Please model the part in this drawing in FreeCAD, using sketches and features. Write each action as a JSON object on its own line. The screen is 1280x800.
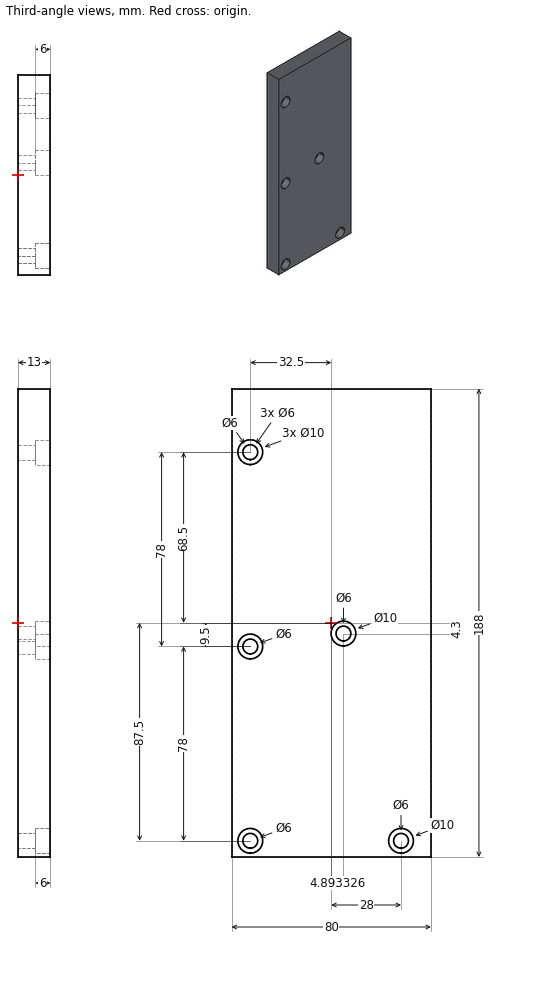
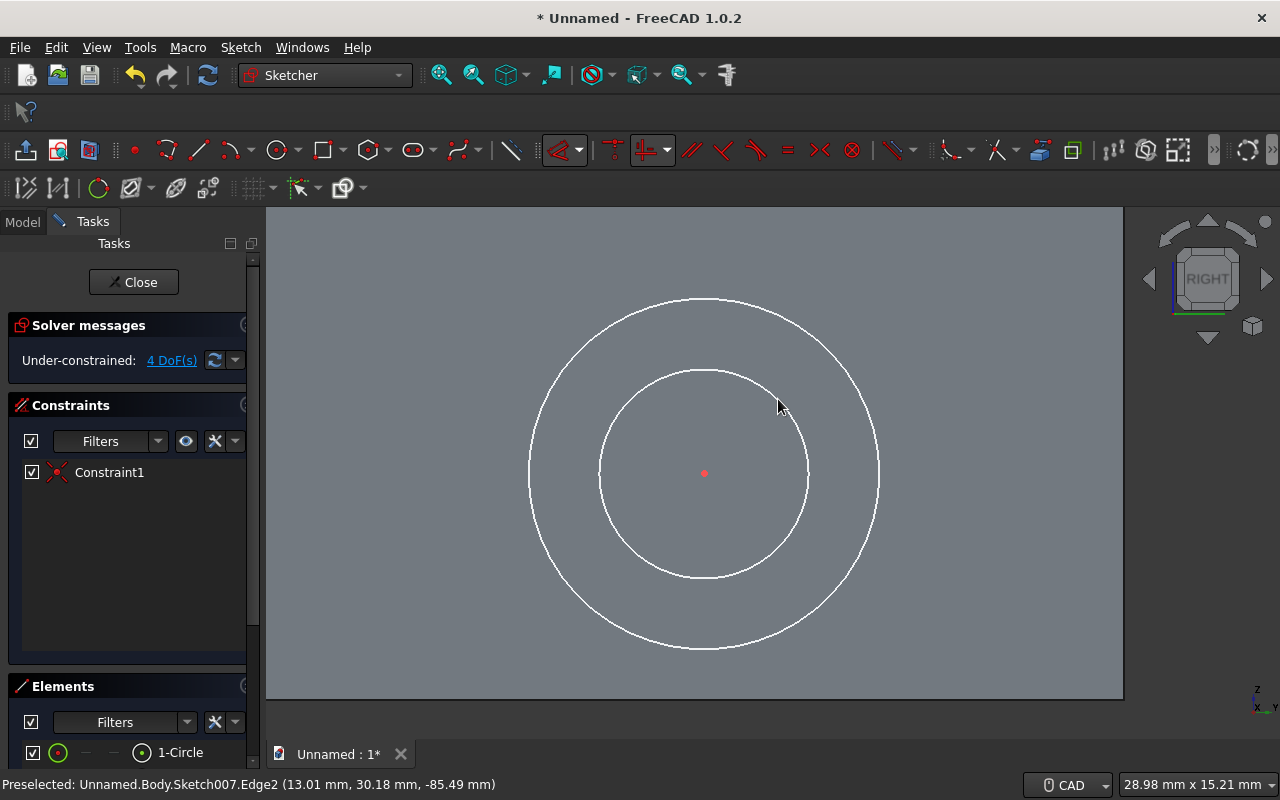
{"action": "left_click", "coordinate": [828, 350]}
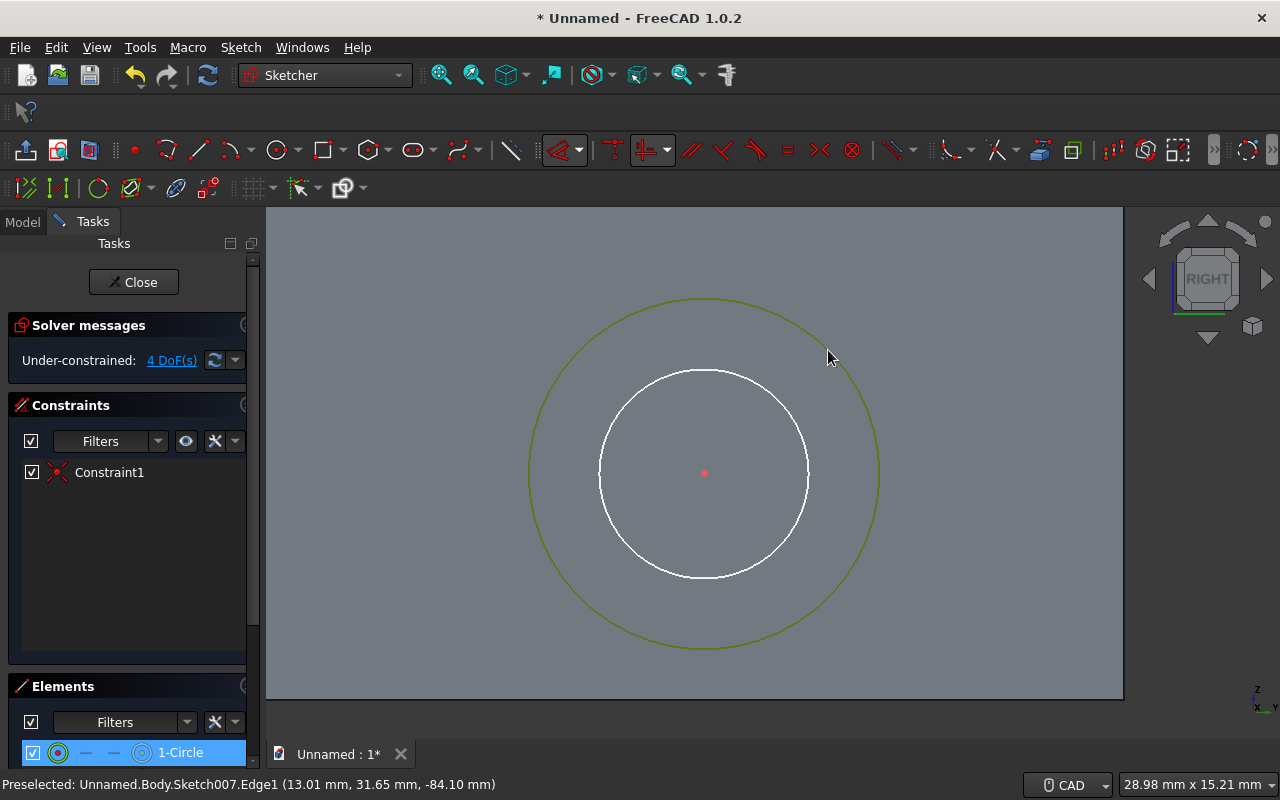
{"action": "left_click", "coordinate": [582, 150]}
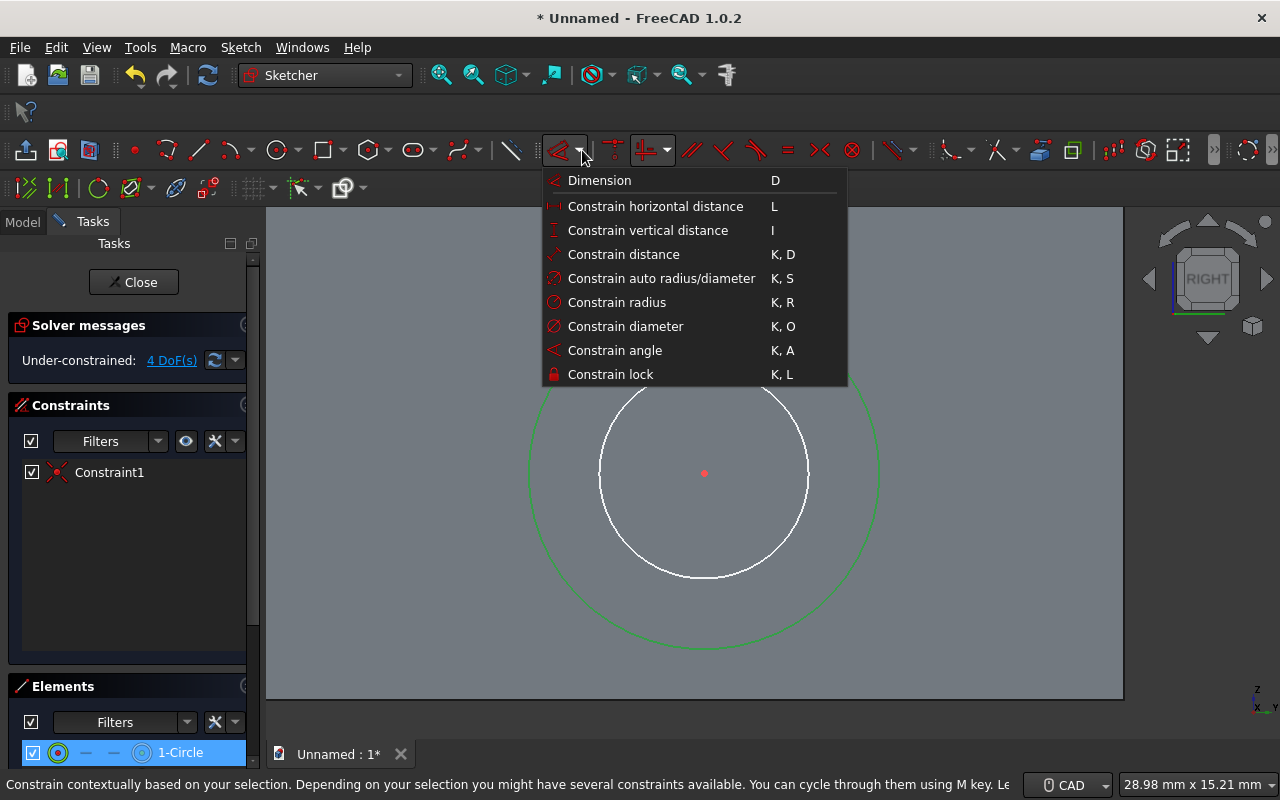
{"action": "left_click", "coordinate": [695, 326]}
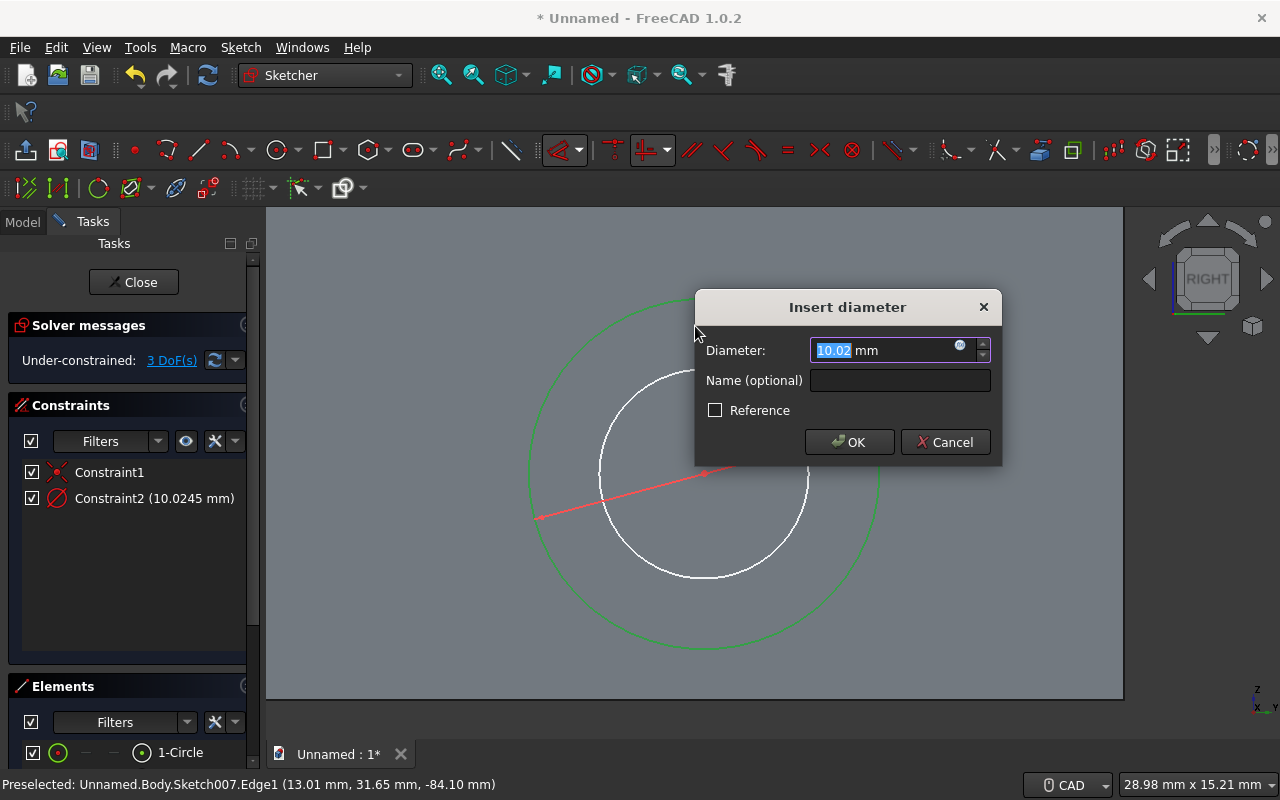
{"action": "type", "text": "10"}
{"action": "key", "text": "Return"}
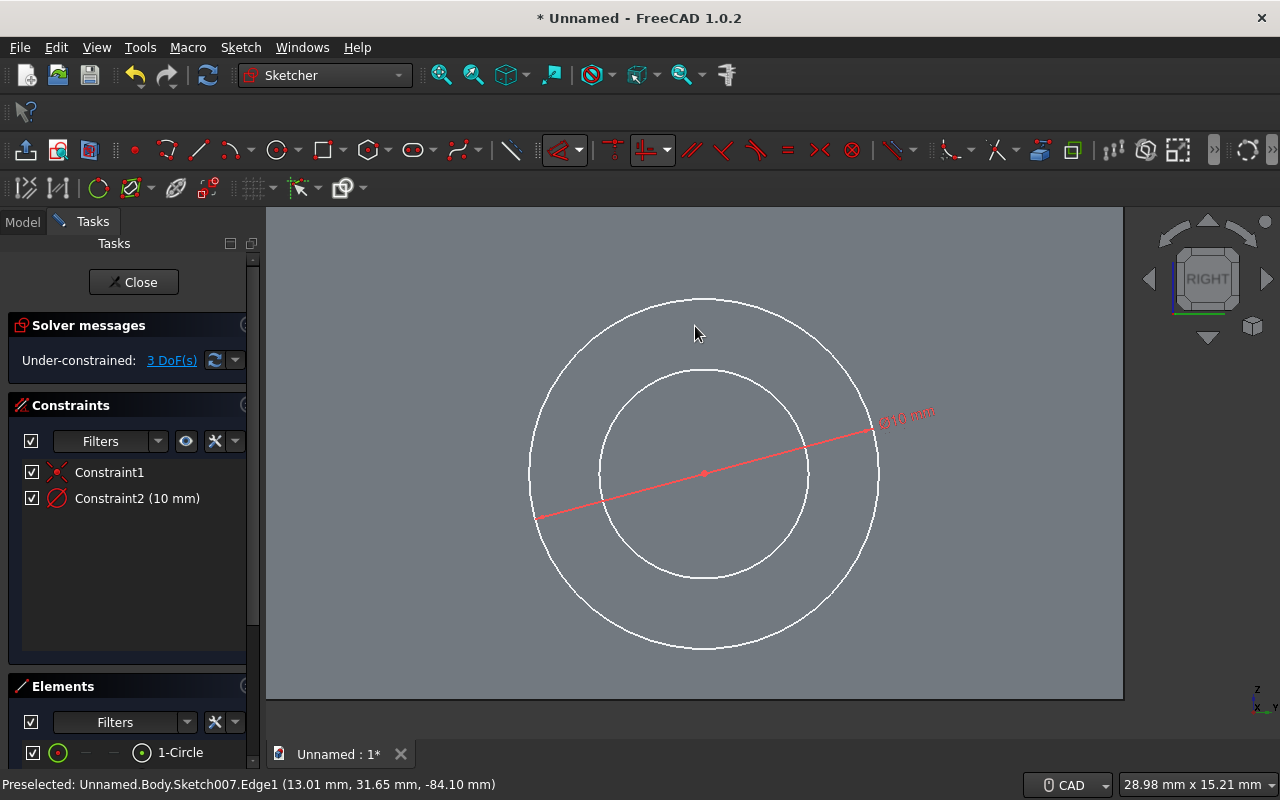
{"action": "left_click", "coordinate": [778, 400]}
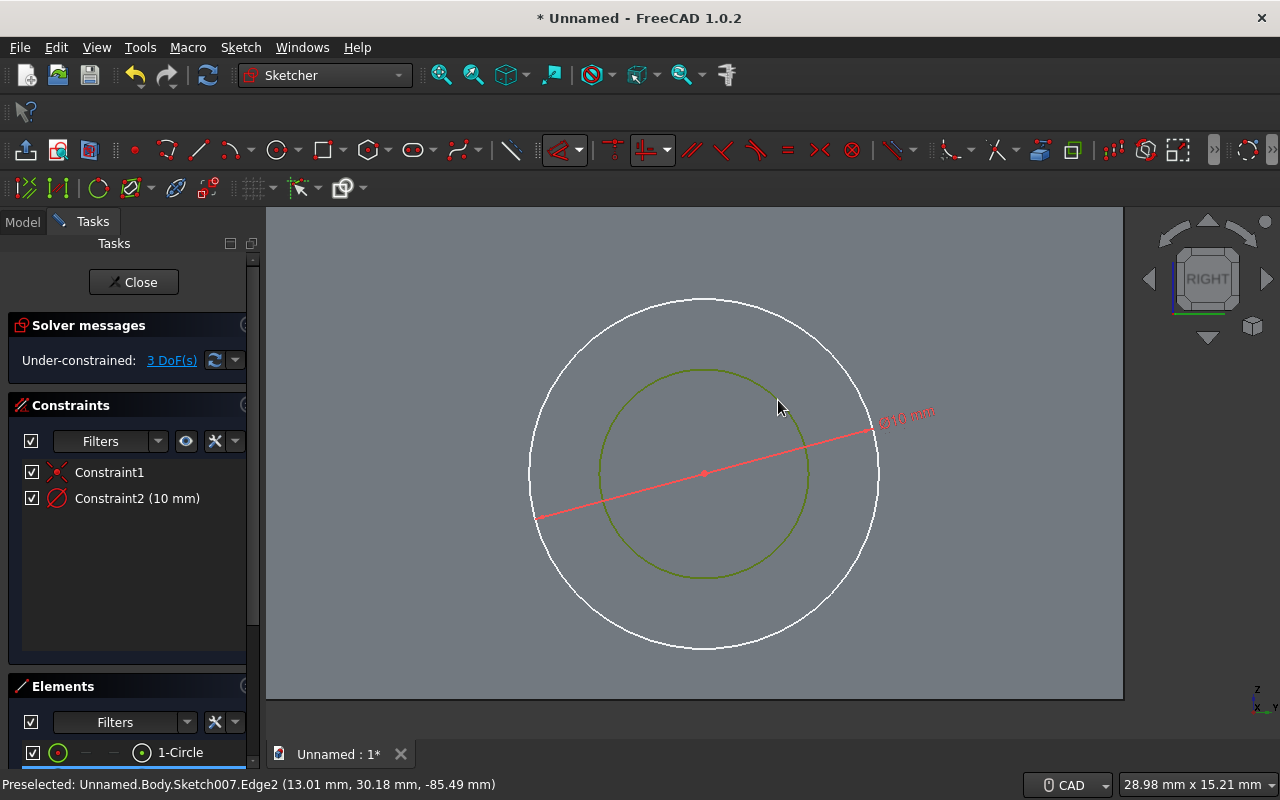
{"action": "key", "text": "k o"}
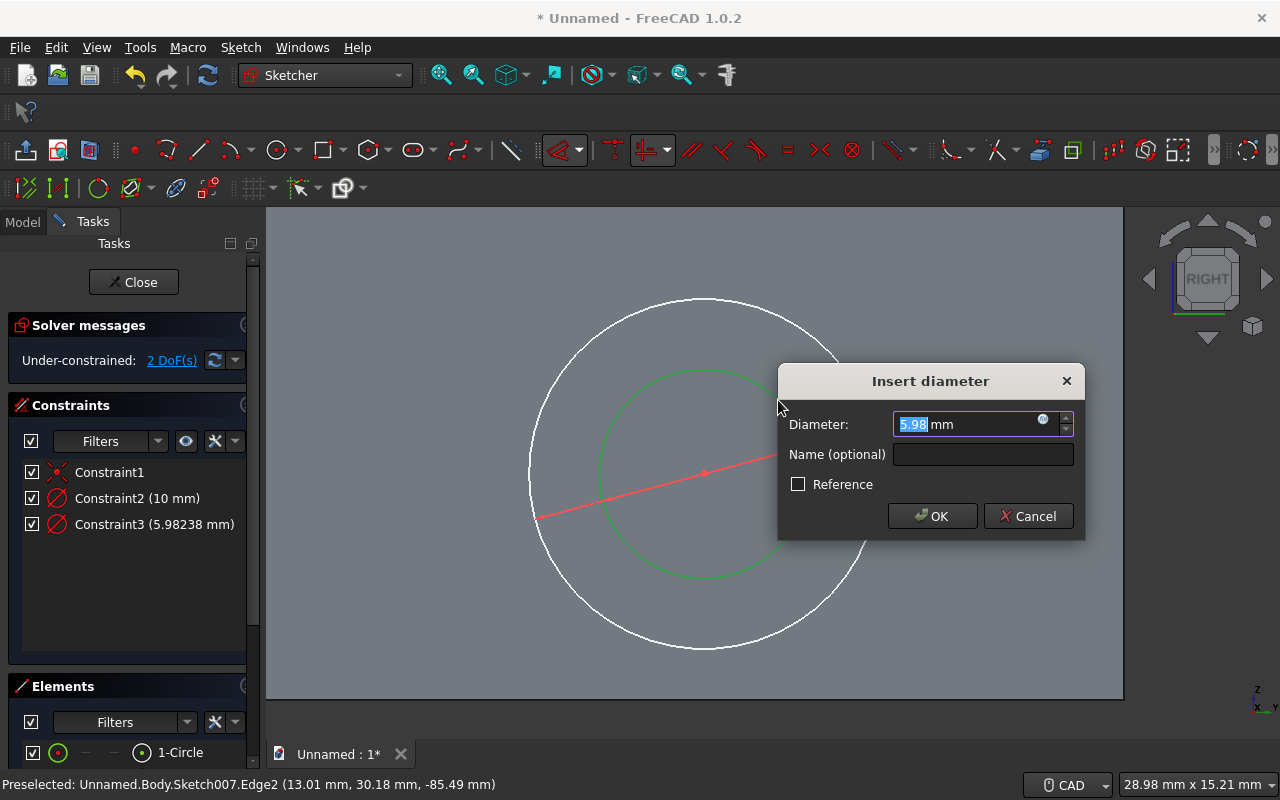
{"action": "type", "text": "6"}
{"action": "key", "text": "Return"}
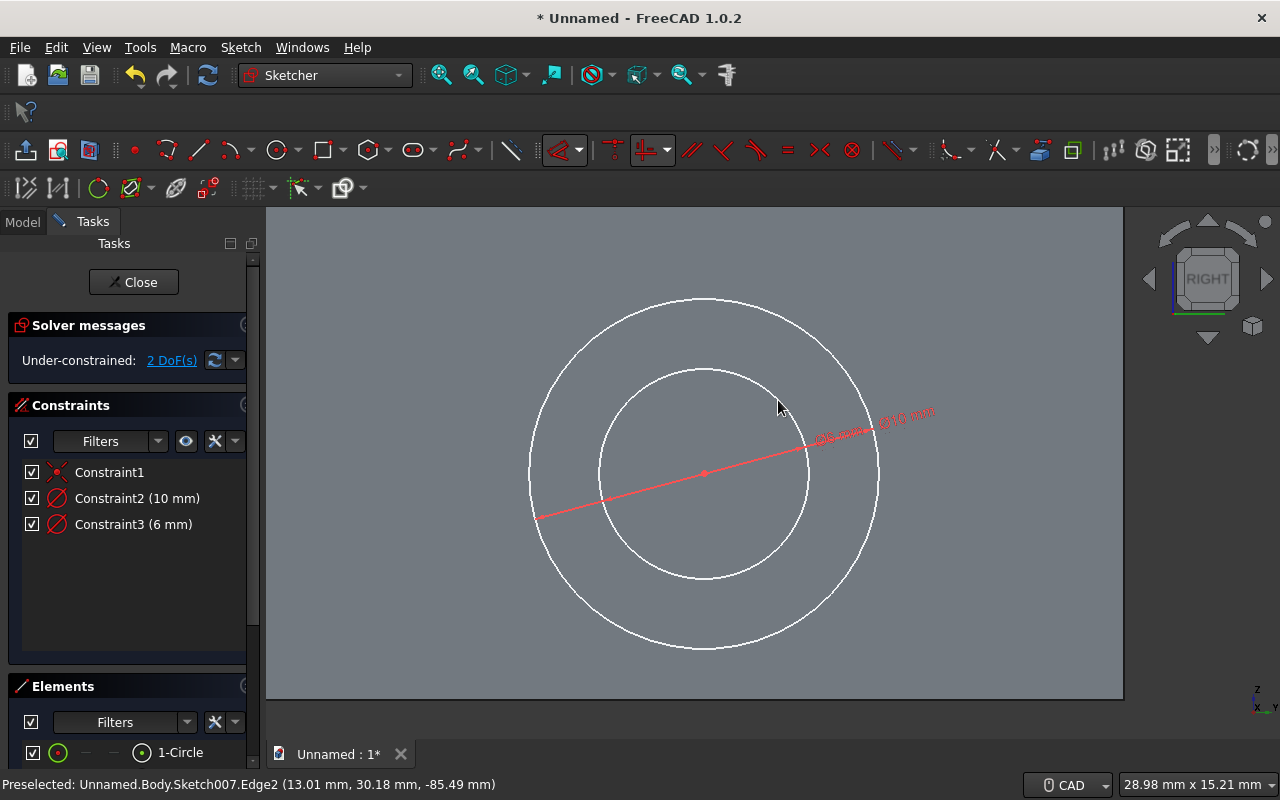
{"action": "left_click", "coordinate": [704, 474]}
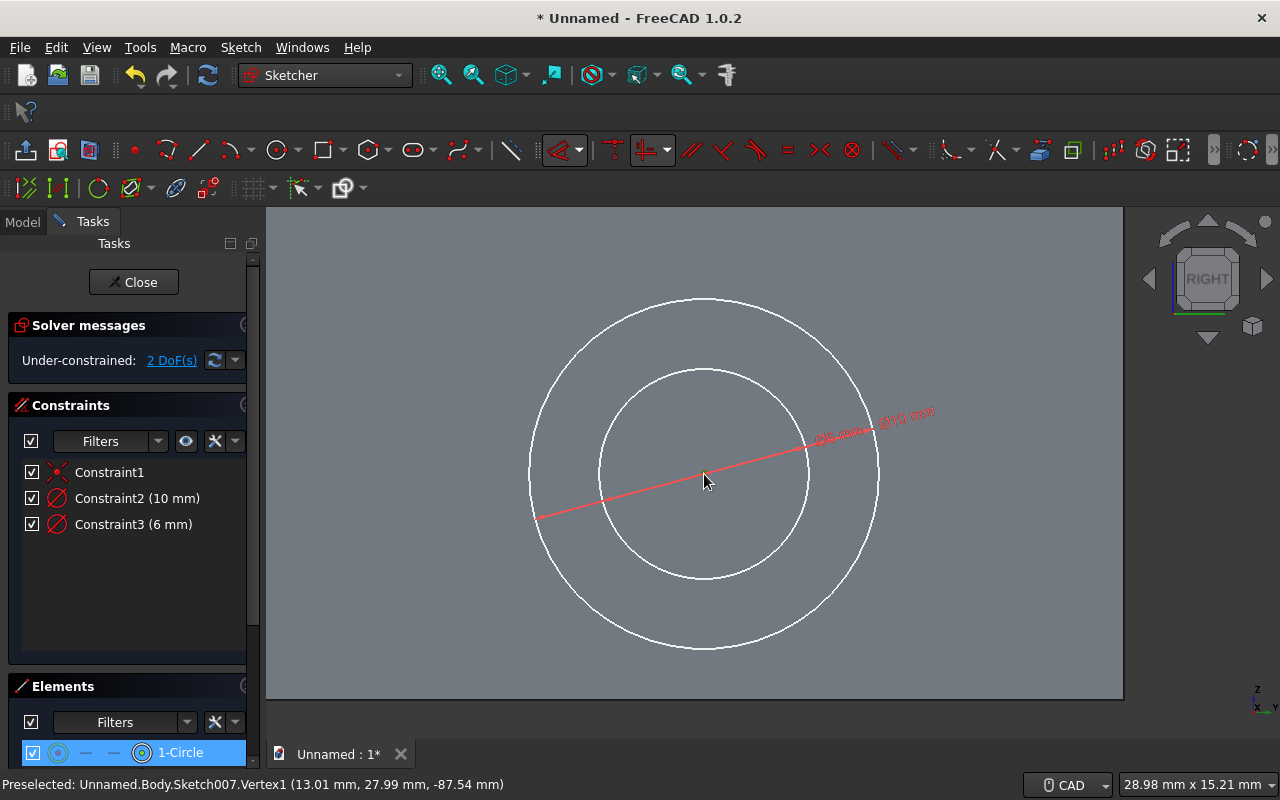
{"action": "left_click", "coordinate": [582, 150]}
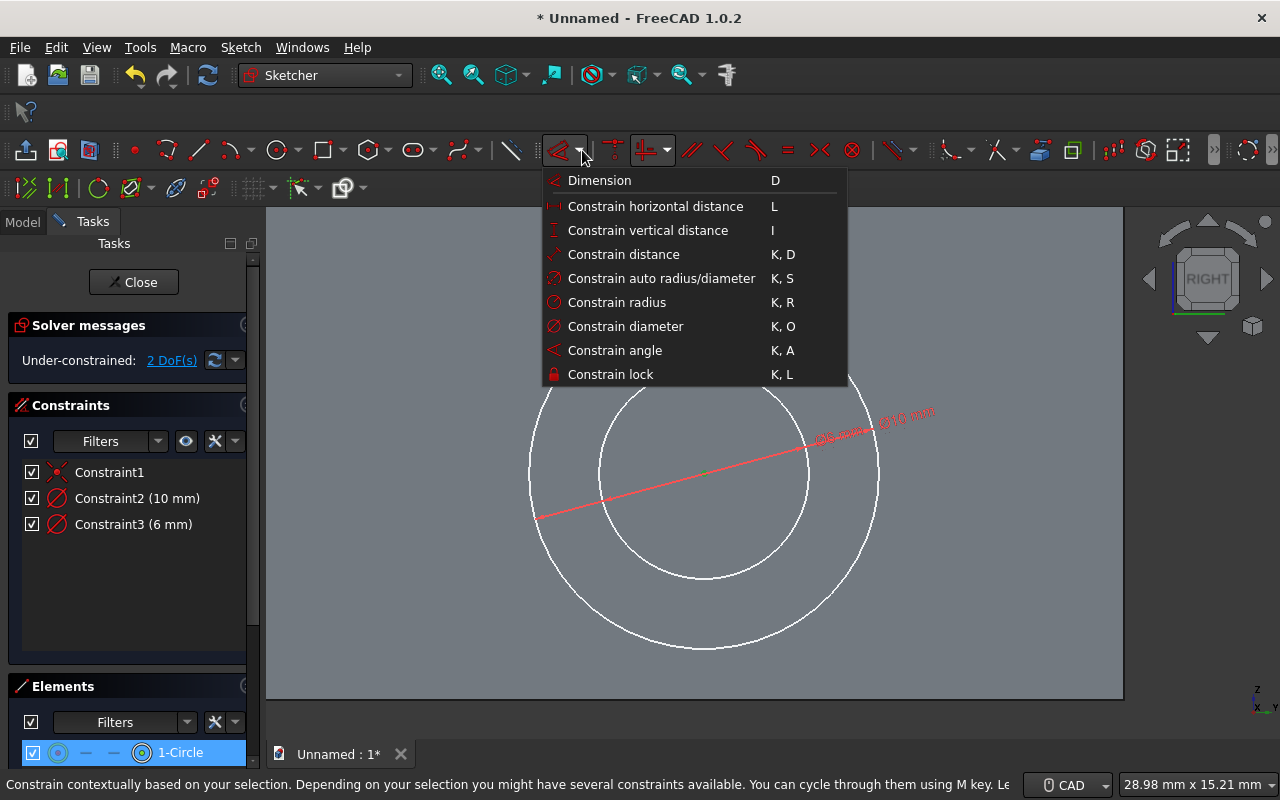
{"action": "left_click", "coordinate": [695, 206]}